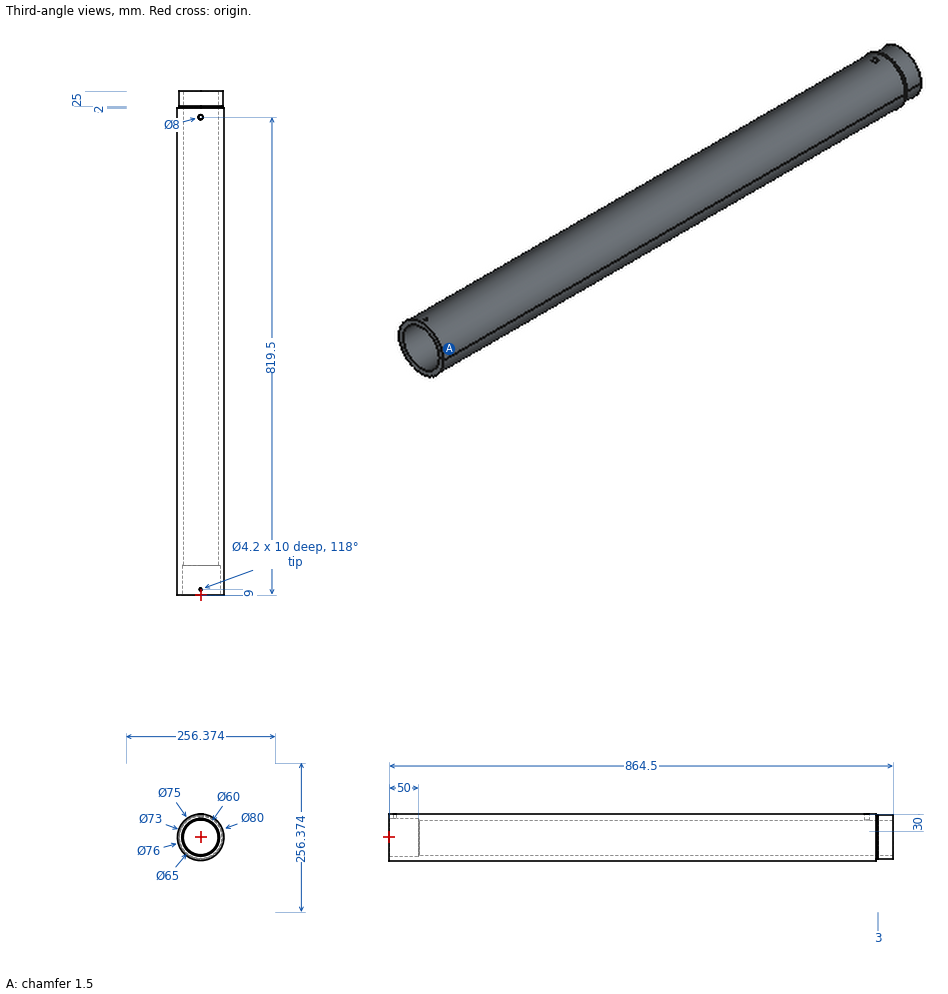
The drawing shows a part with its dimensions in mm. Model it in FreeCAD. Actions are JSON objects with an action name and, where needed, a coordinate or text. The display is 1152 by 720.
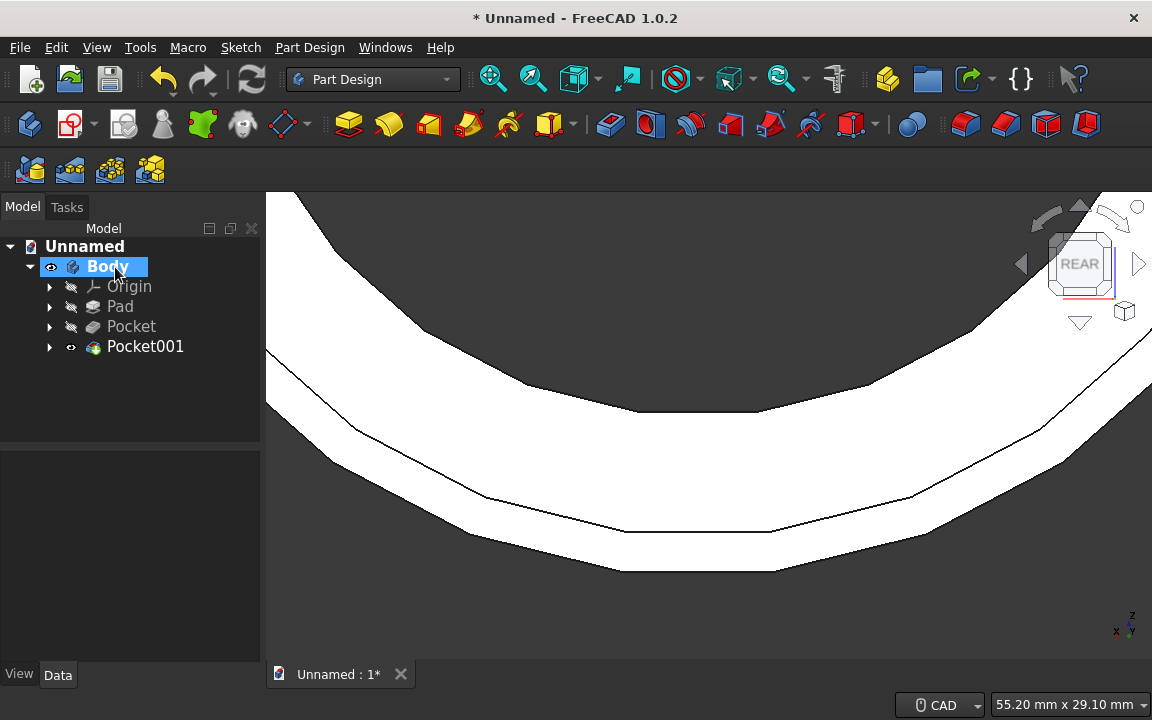
{"action": "key", "text": "v f"}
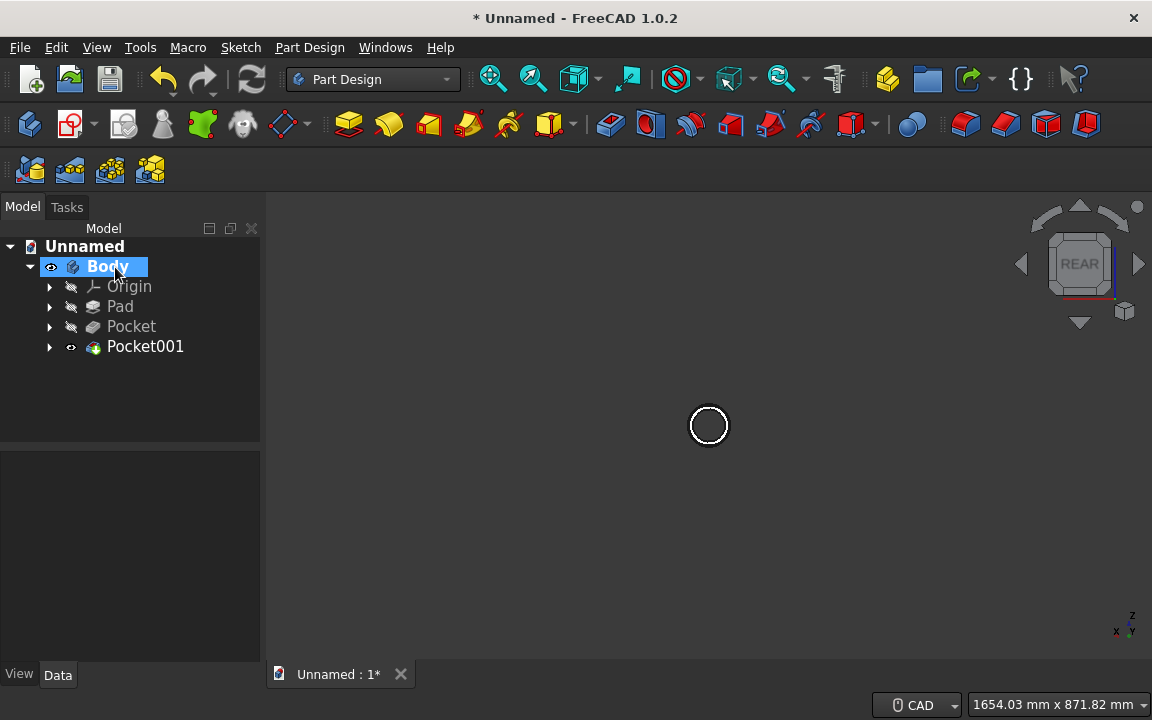
{"action": "scroll", "coordinate": [704, 445], "scroll_direction": "up", "scroll_amount": 15}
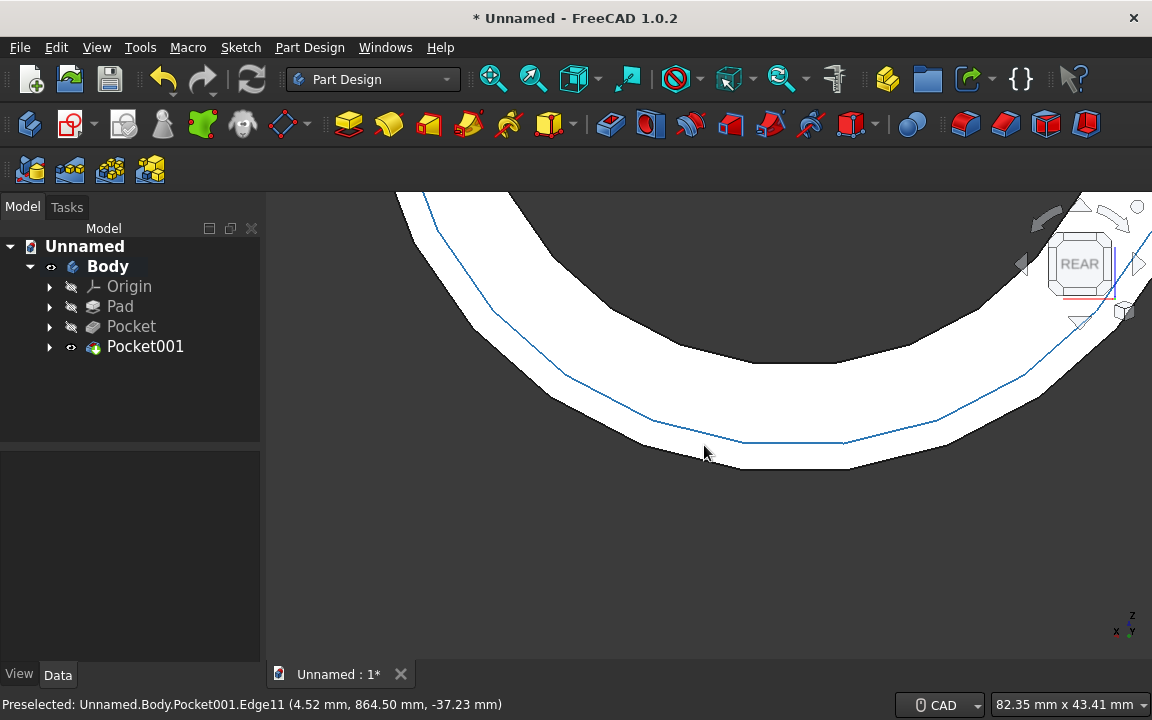
{"action": "left_click", "coordinate": [689, 446]}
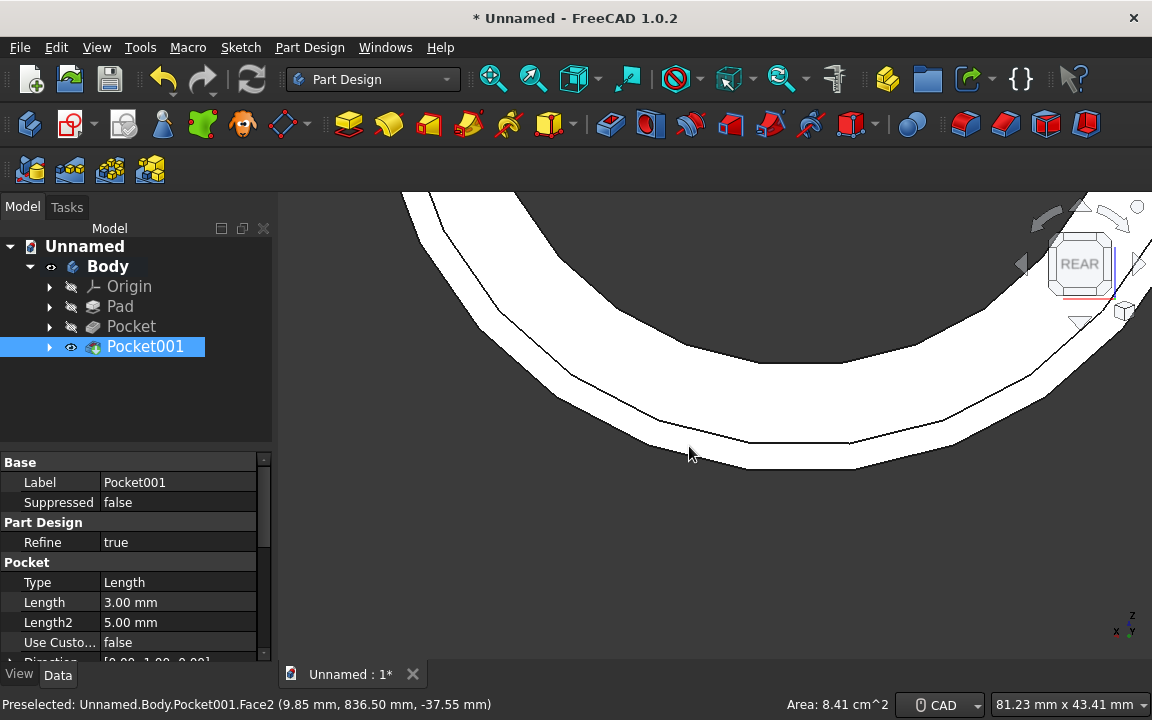
{"action": "left_click", "coordinate": [70, 124]}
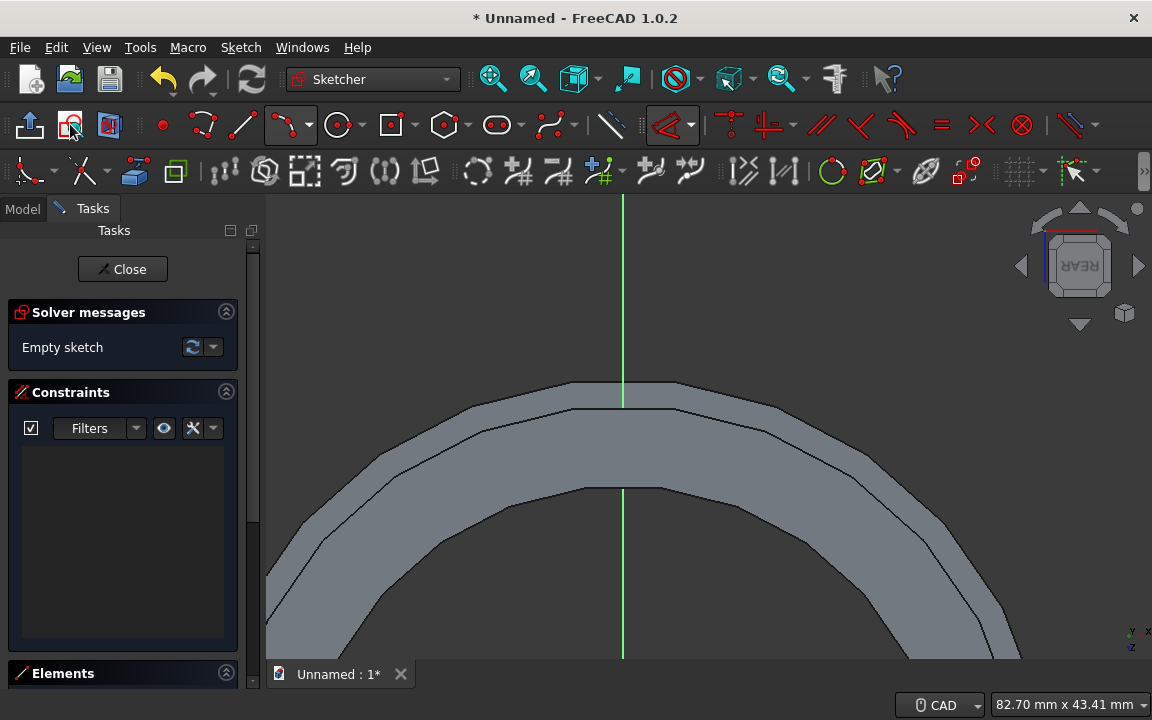
{"action": "left_click", "coordinate": [110, 126]}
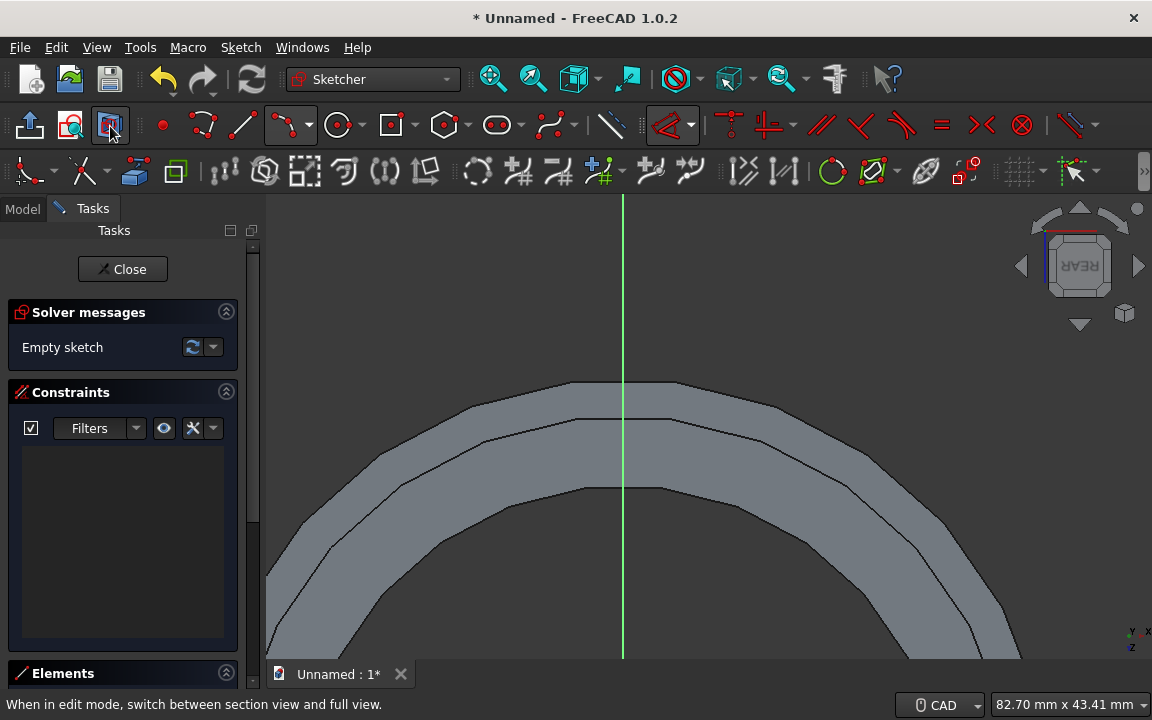
{"action": "scroll", "coordinate": [643, 379], "scroll_direction": "down", "scroll_amount": 11}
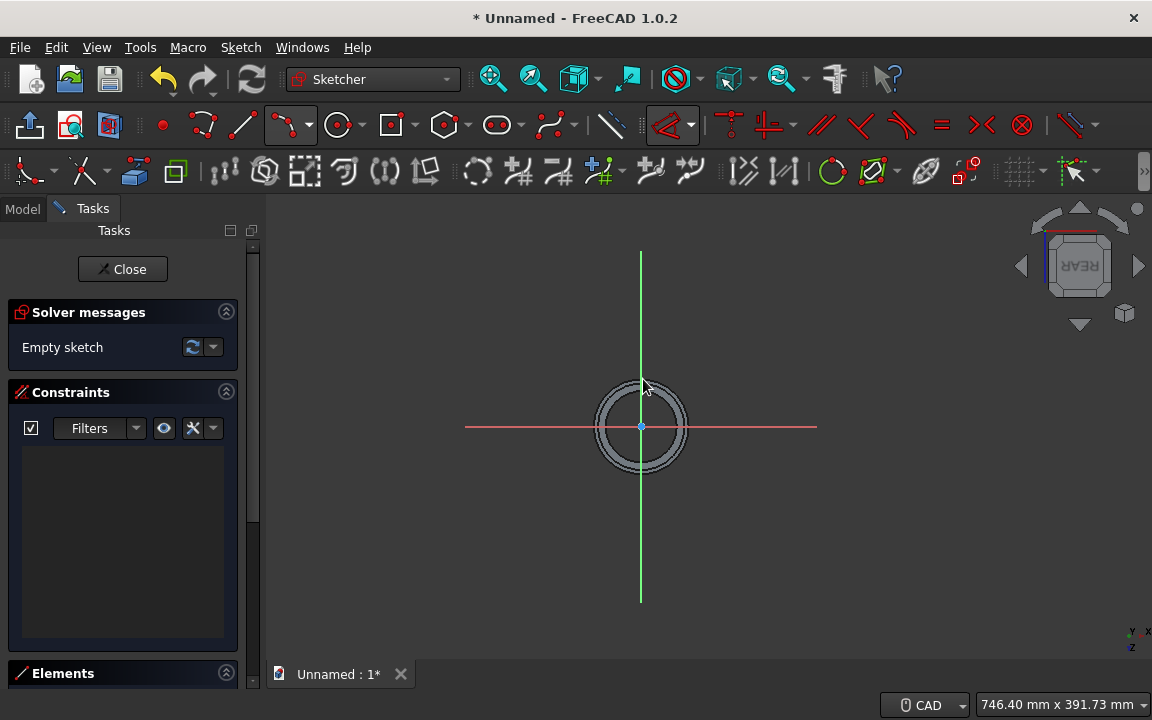
{"action": "left_click", "coordinate": [392, 126]}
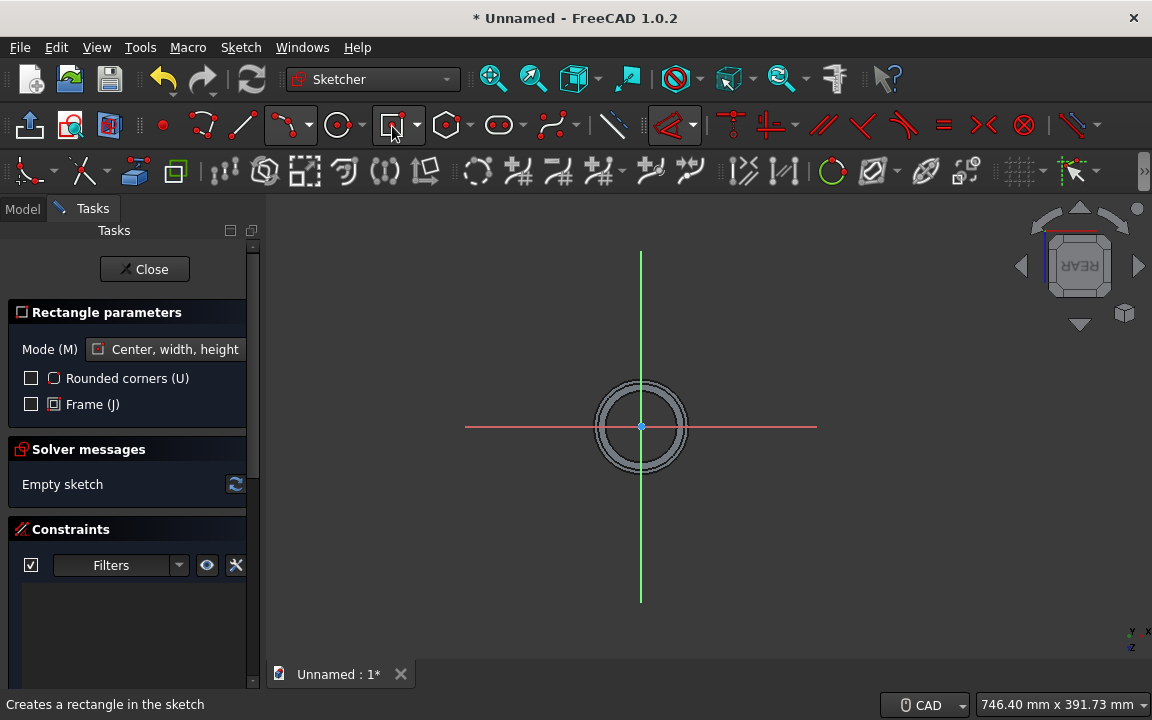
{"action": "left_click", "coordinate": [641, 427]}
{"action": "mouse_move", "coordinate": [793, 275]}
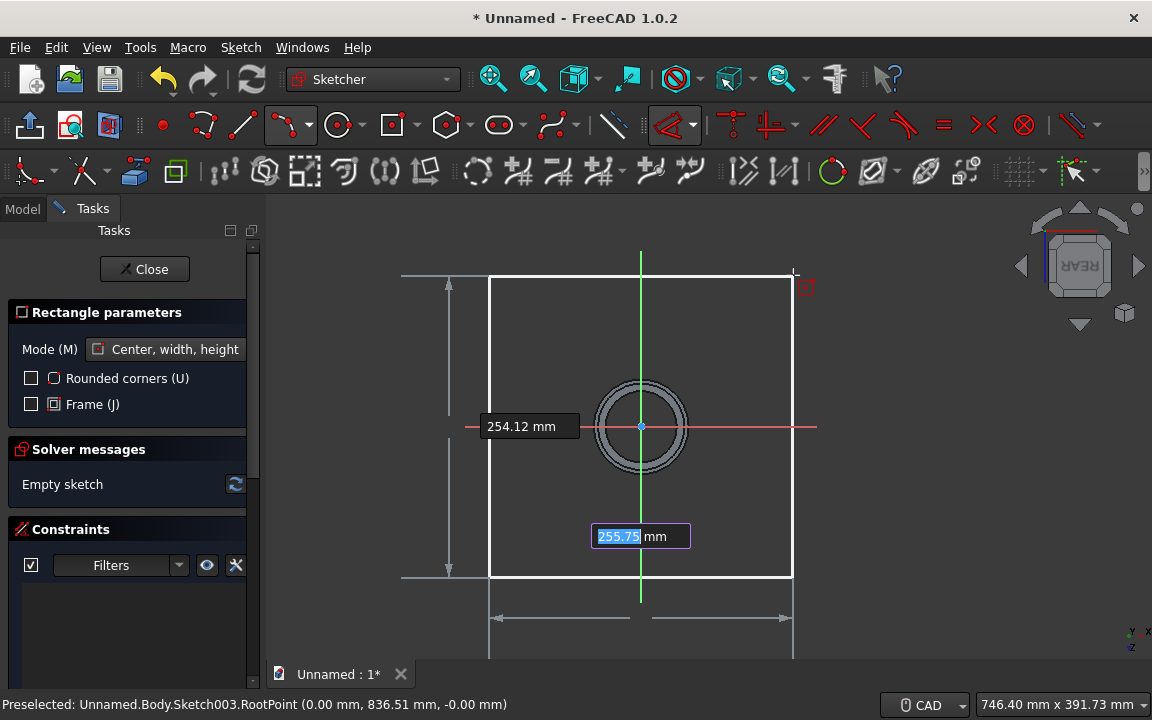
{"action": "type", "text": "256.374"}
{"action": "key", "text": "Tab"}
{"action": "type", "text": "256.374"}
{"action": "key", "text": "Return"}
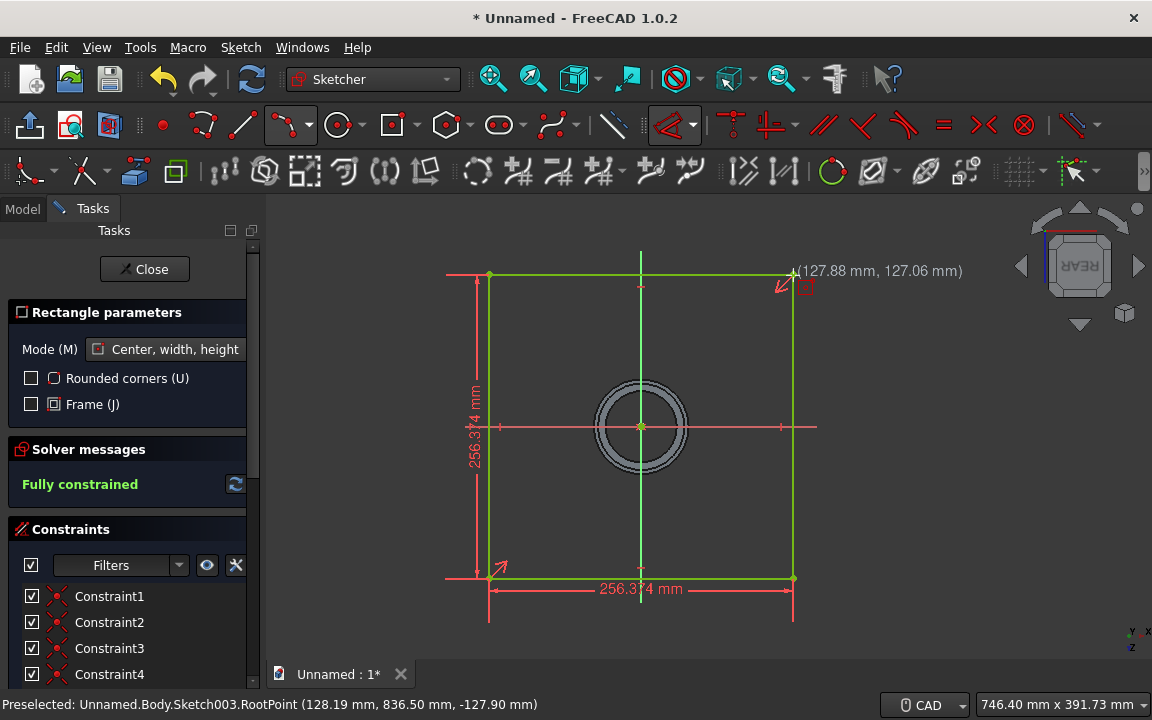
{"action": "left_click", "coordinate": [338, 126]}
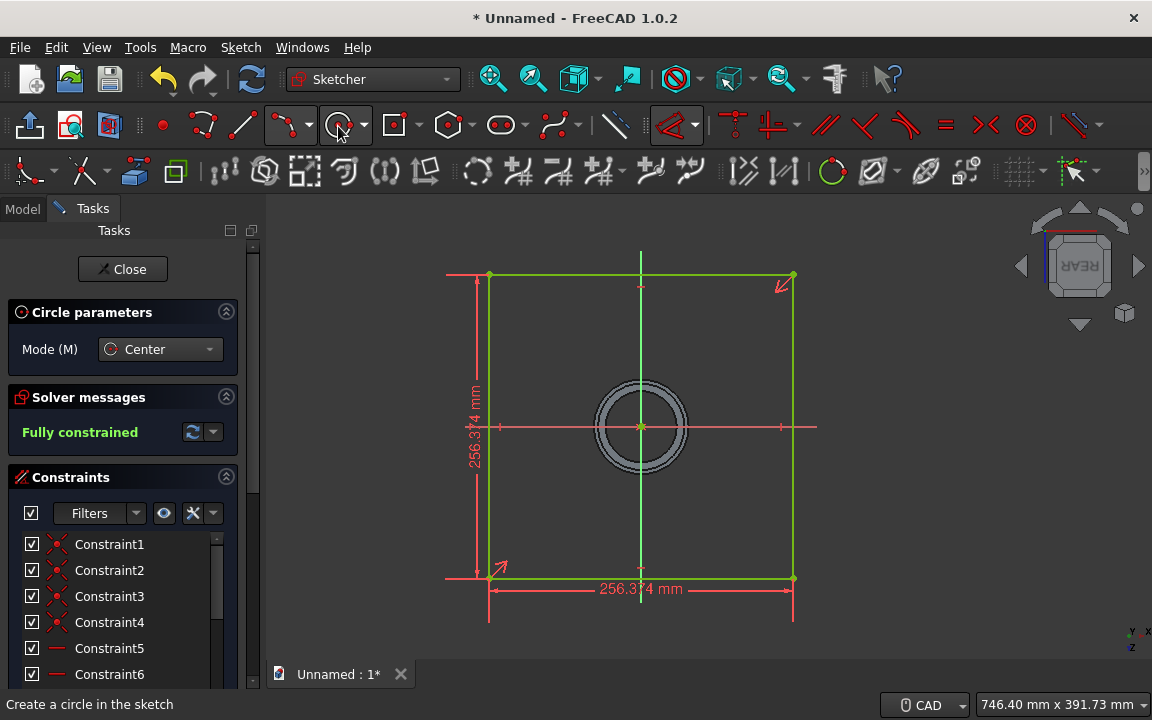
{"action": "left_click", "coordinate": [641, 427]}
{"action": "mouse_move", "coordinate": [673, 395]}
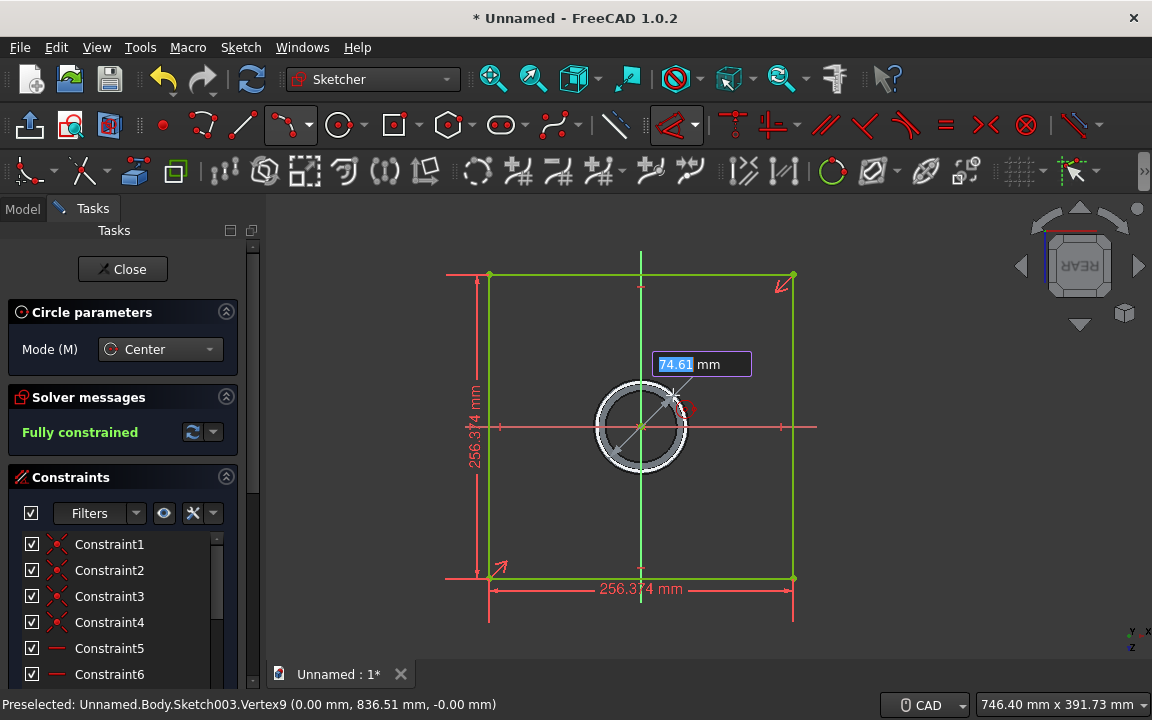
{"action": "type", "text": "76"}
{"action": "key", "text": "Return"}
{"action": "key", "text": "Escape"}